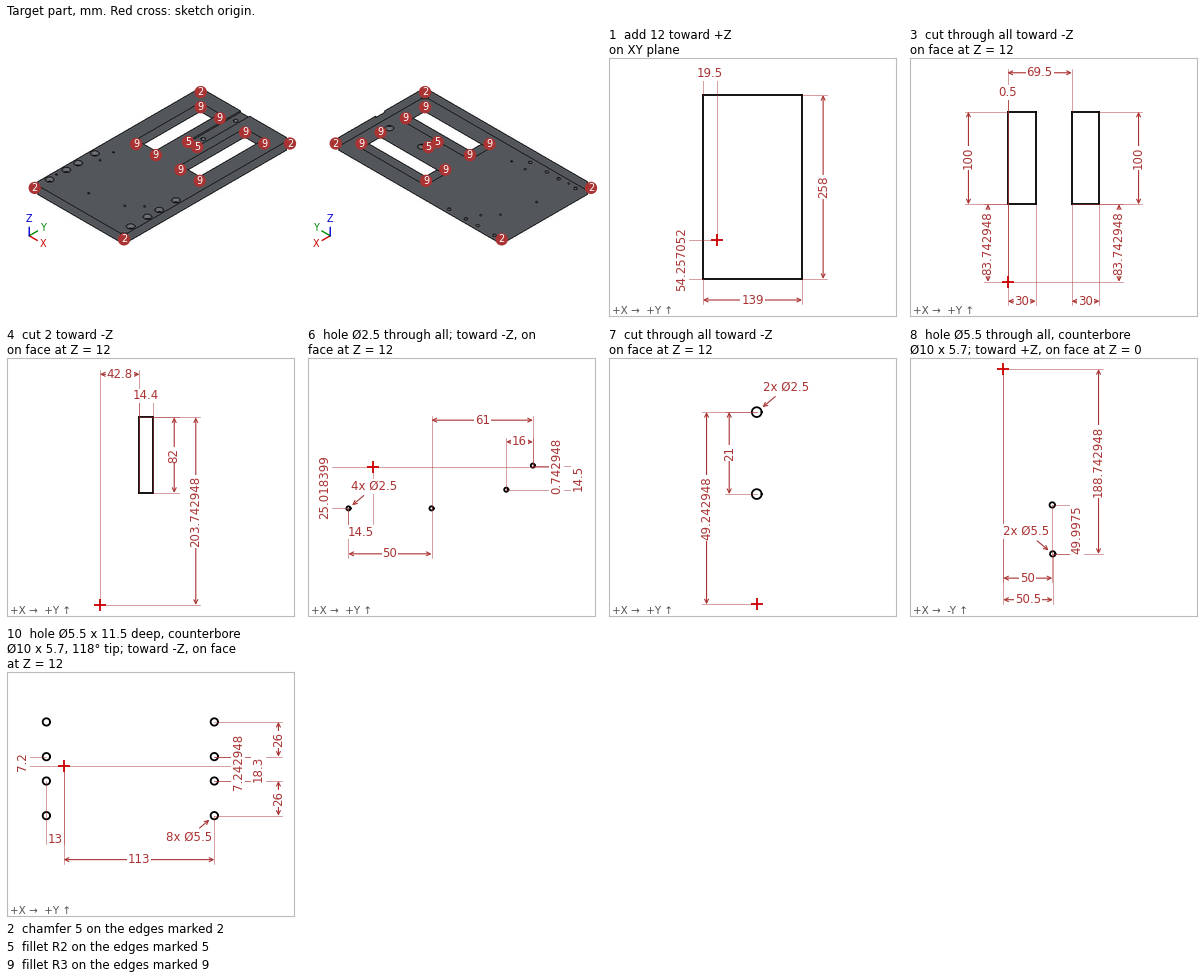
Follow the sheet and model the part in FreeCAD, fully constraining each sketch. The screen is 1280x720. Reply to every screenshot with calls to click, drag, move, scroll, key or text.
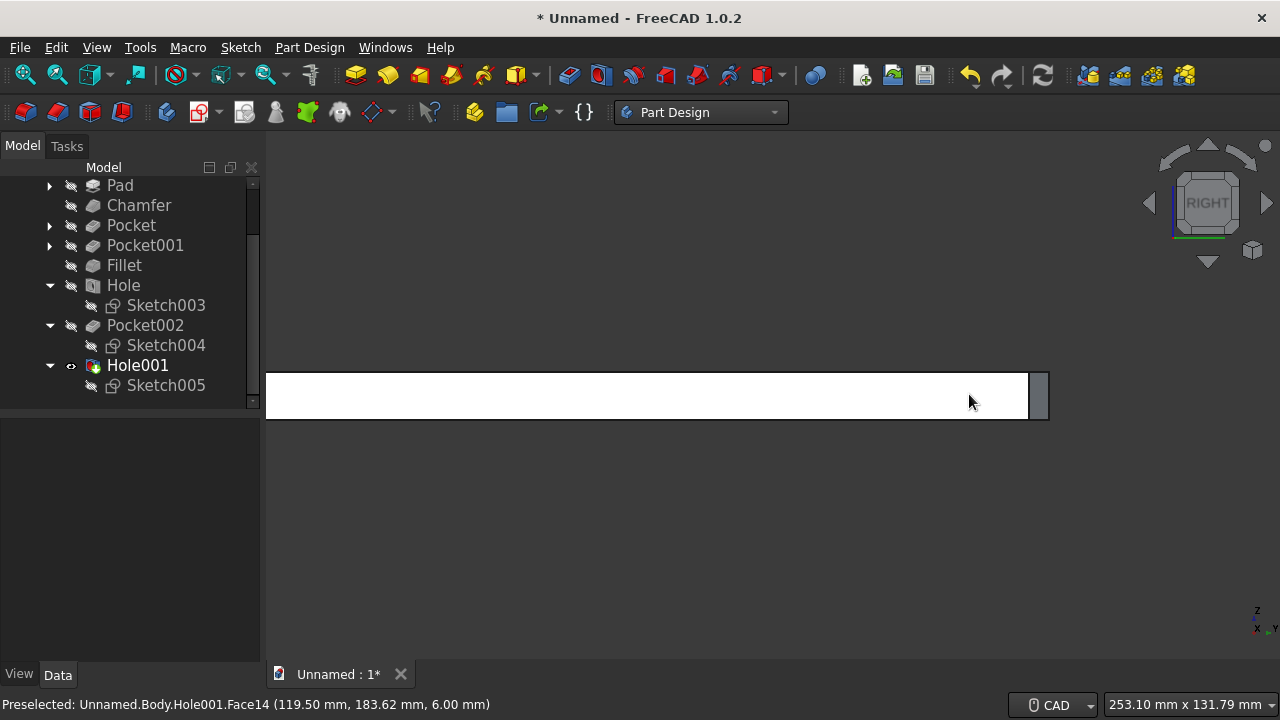
key(v)
key(f)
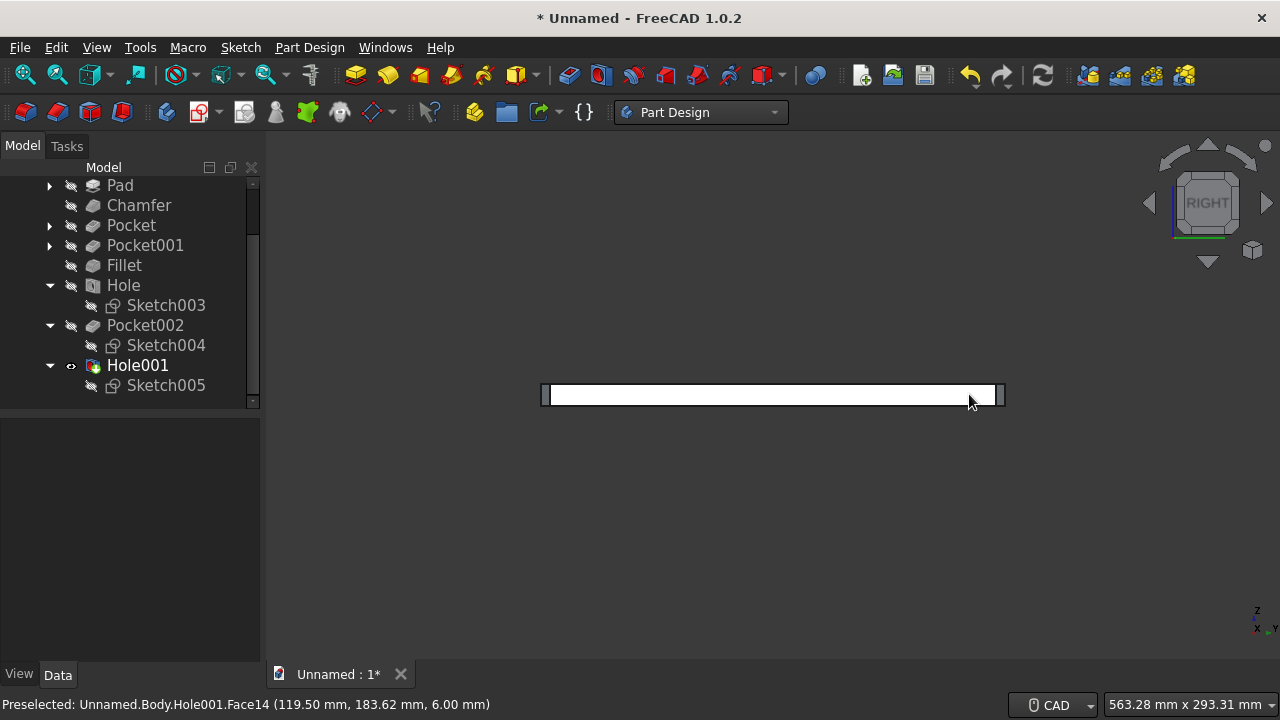
key(5)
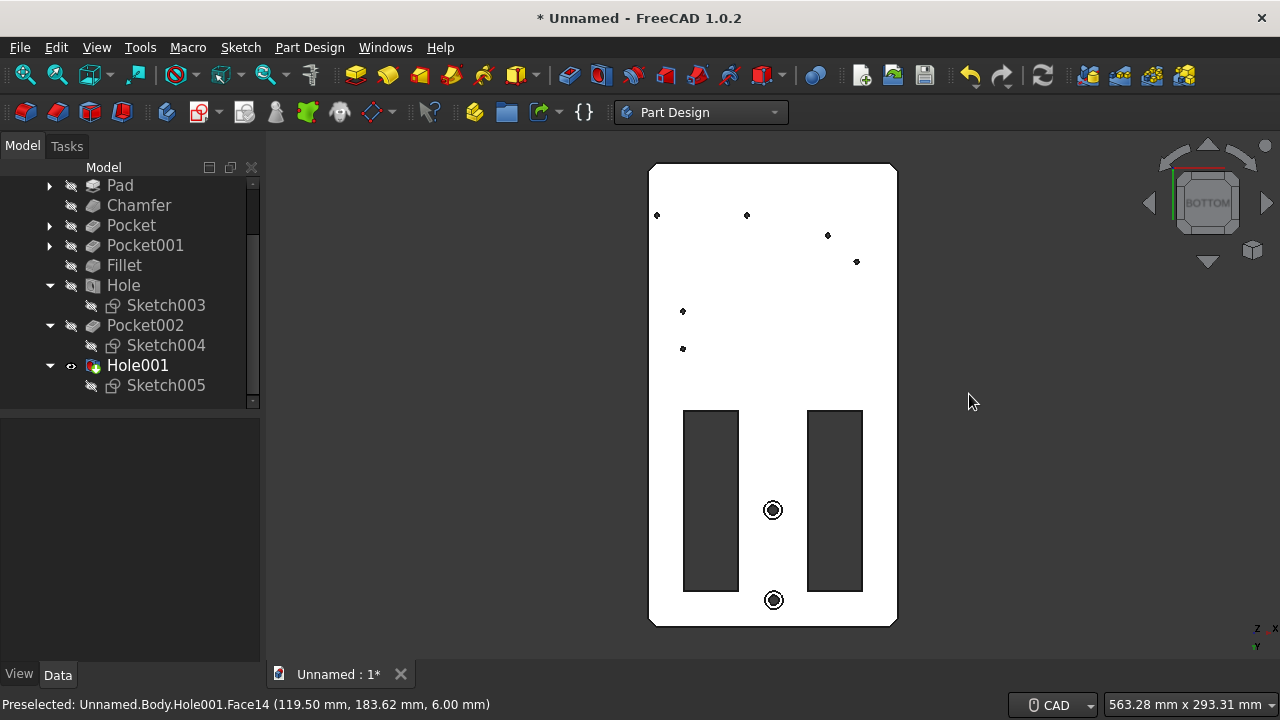
scroll(862, 590, up, 4)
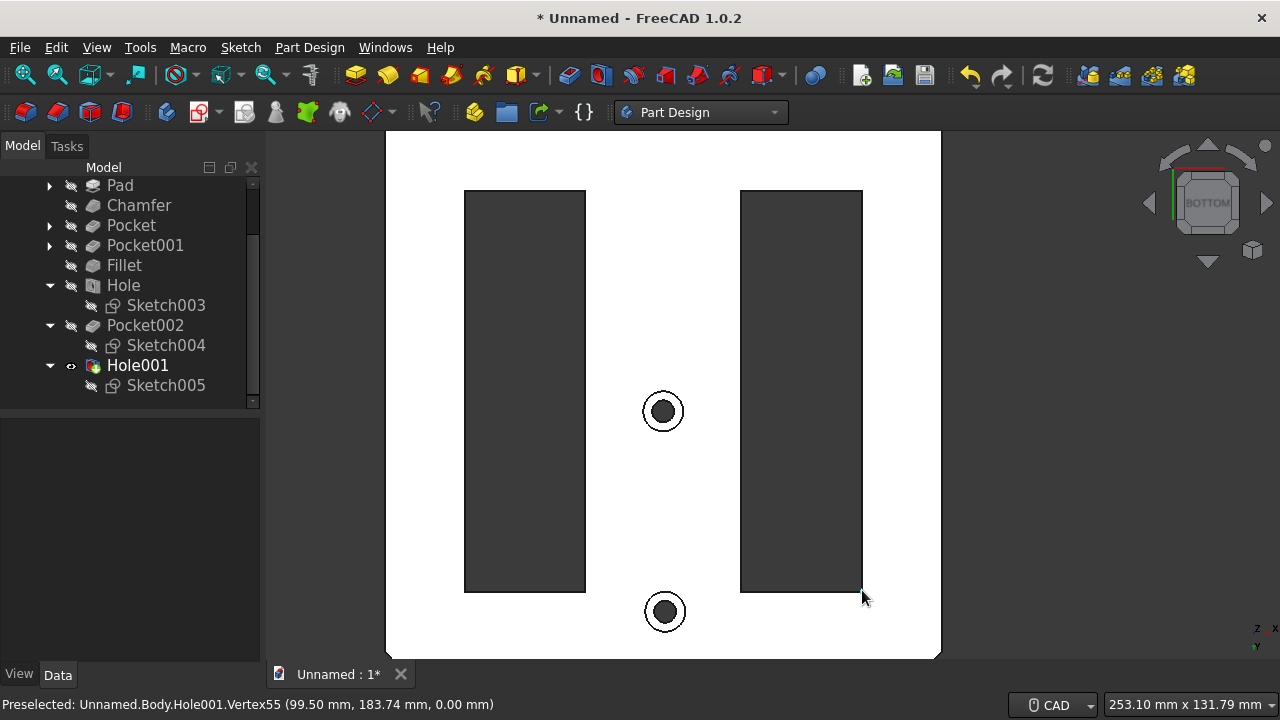
key(v)
key(f)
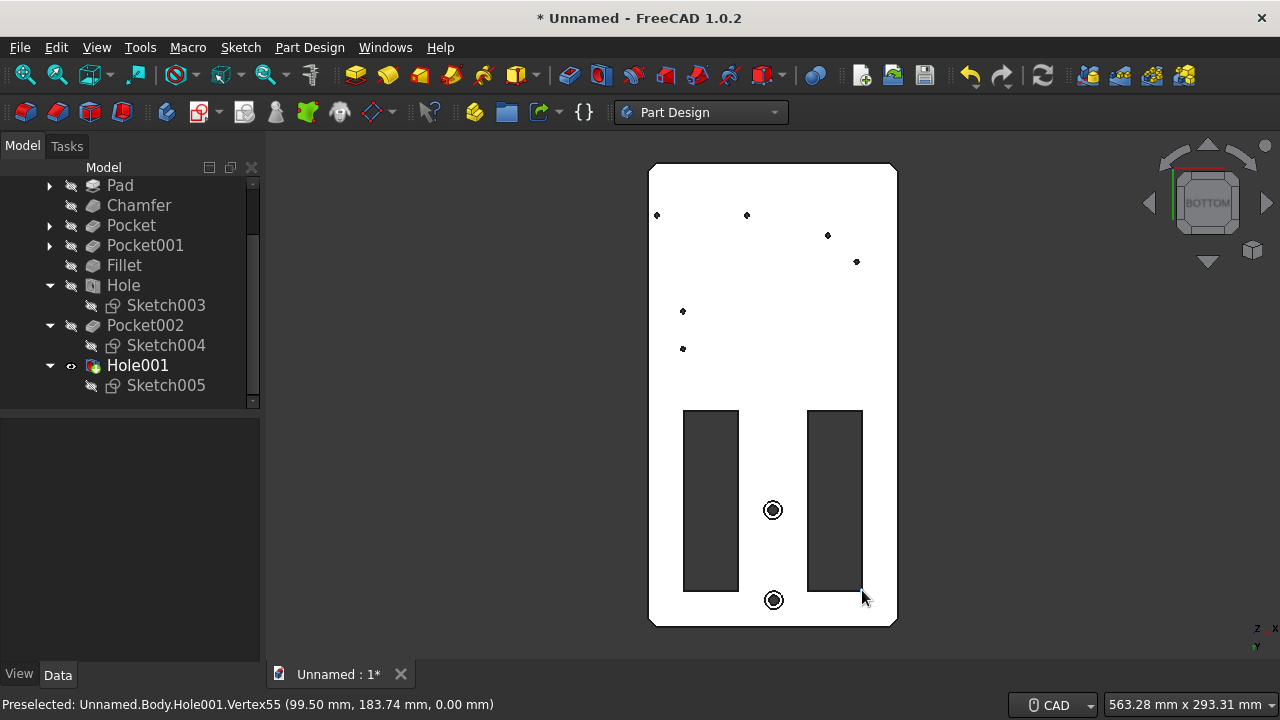
key(4)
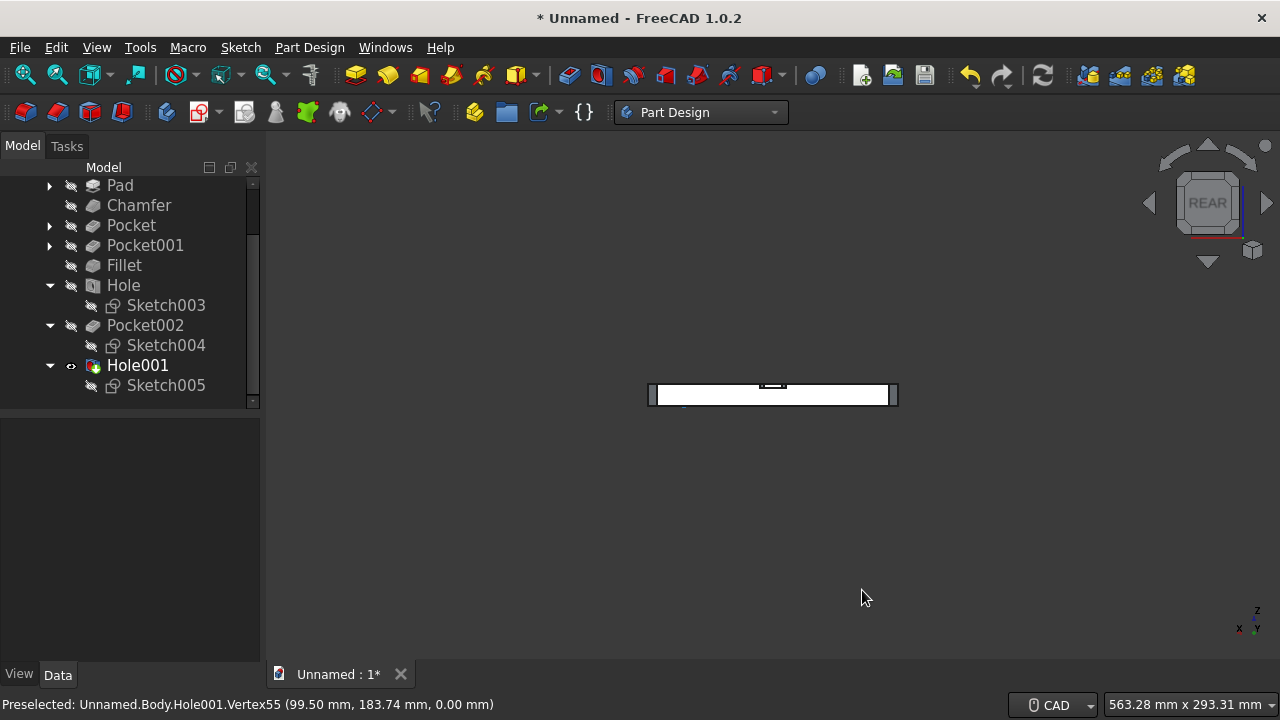
key(v)
key(f)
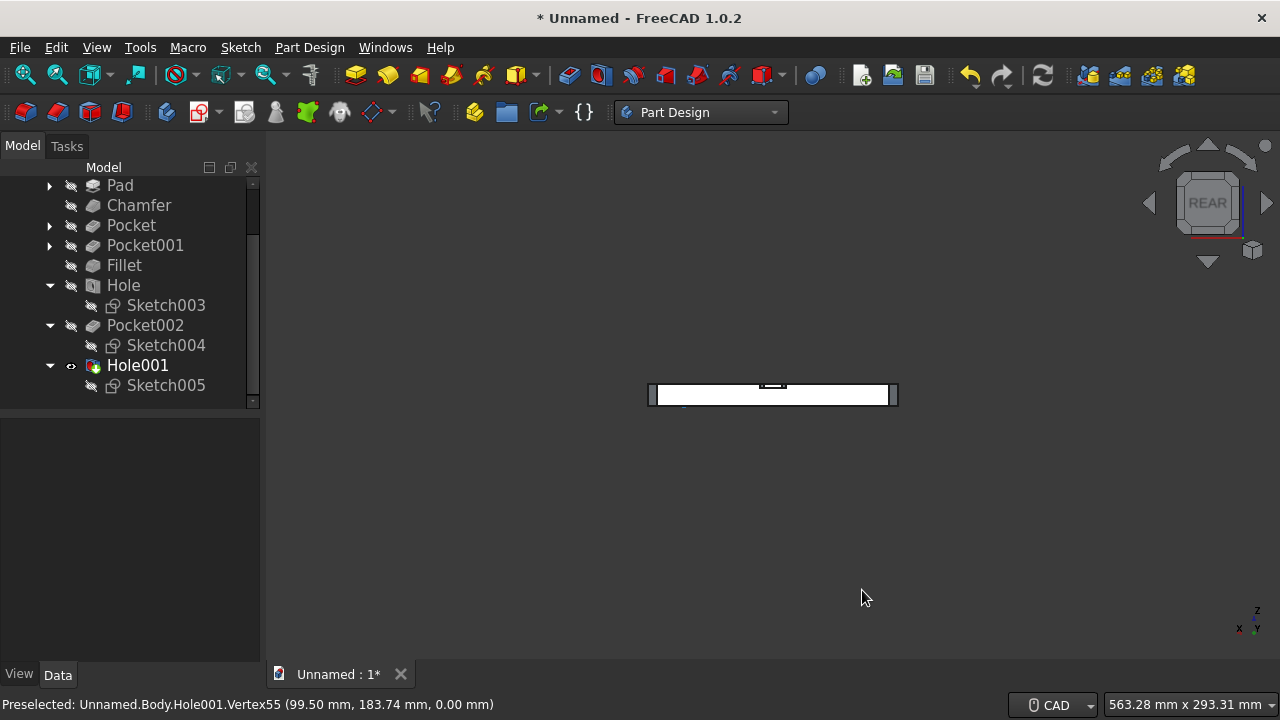
scroll(684, 394, up, 4)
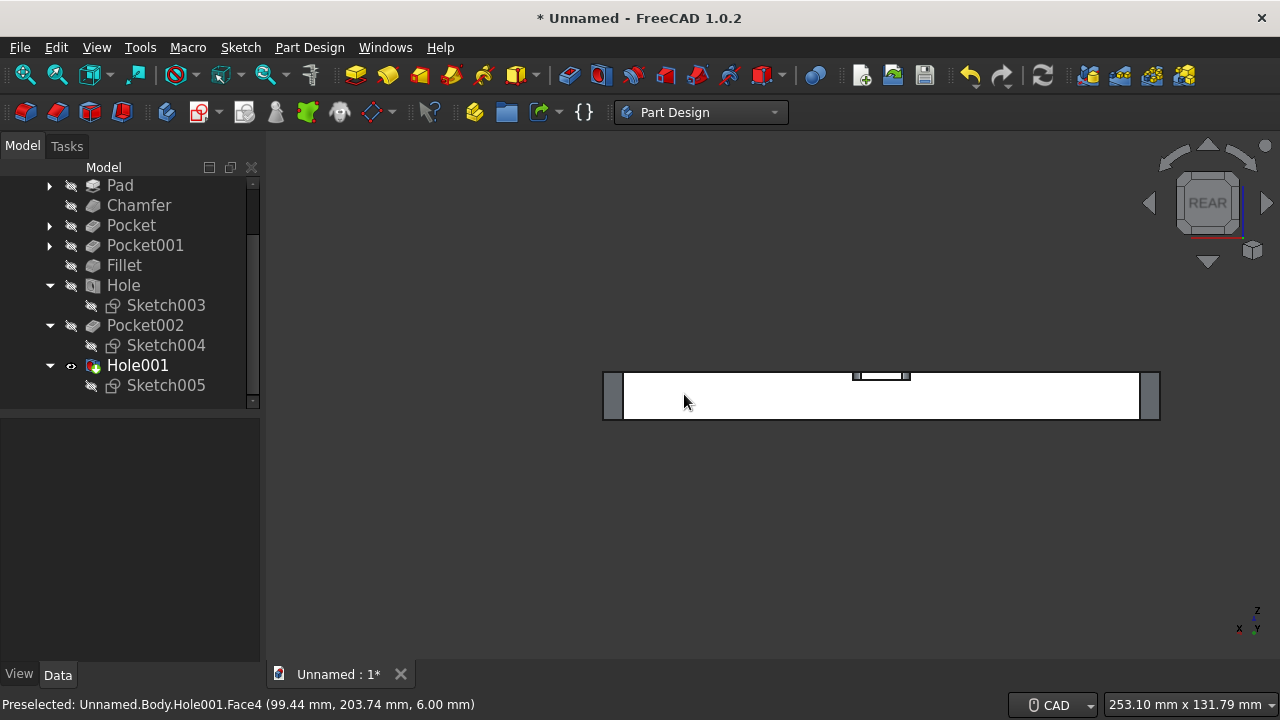
key(v)
key(f)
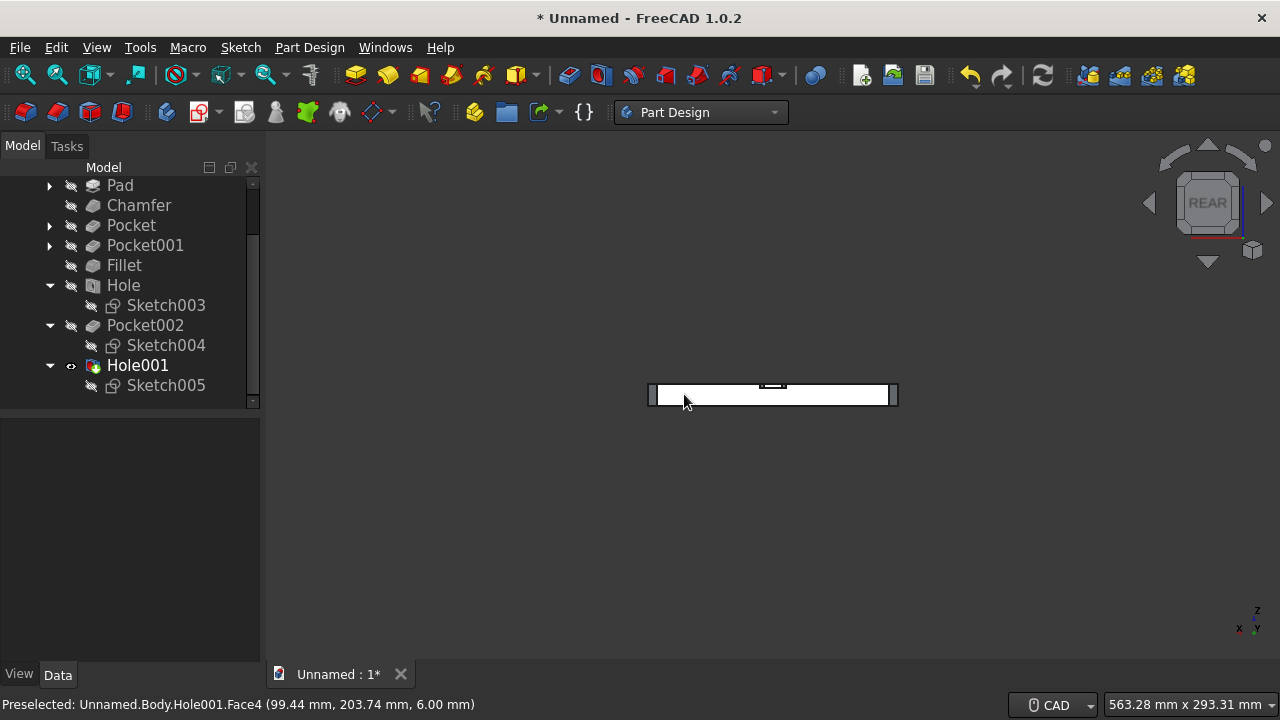
key(6)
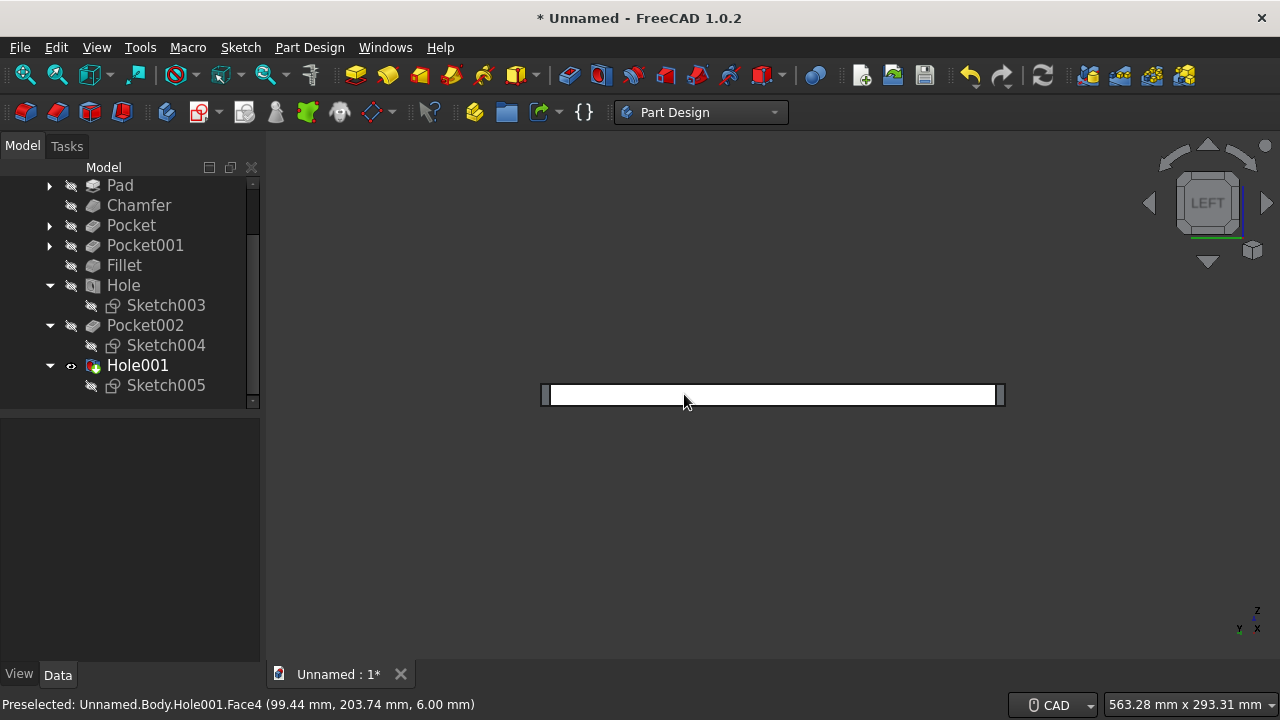
scroll(577, 394, up, 4)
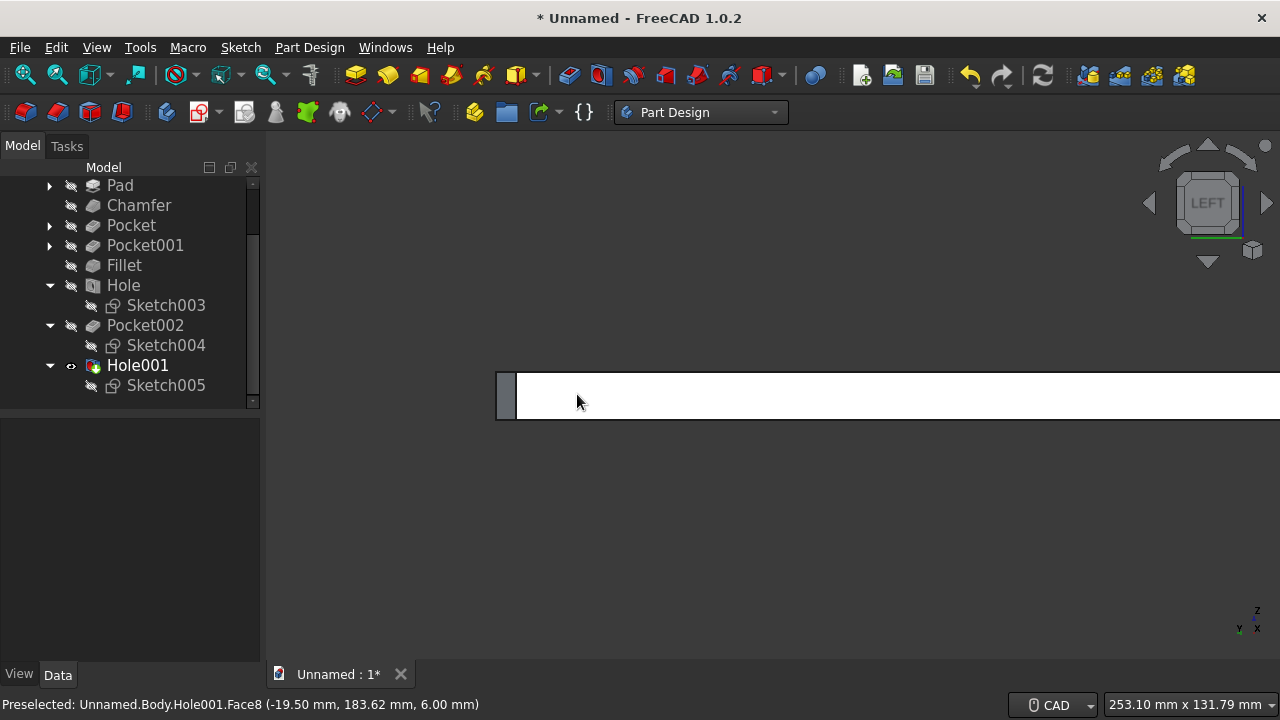
click(26, 76)